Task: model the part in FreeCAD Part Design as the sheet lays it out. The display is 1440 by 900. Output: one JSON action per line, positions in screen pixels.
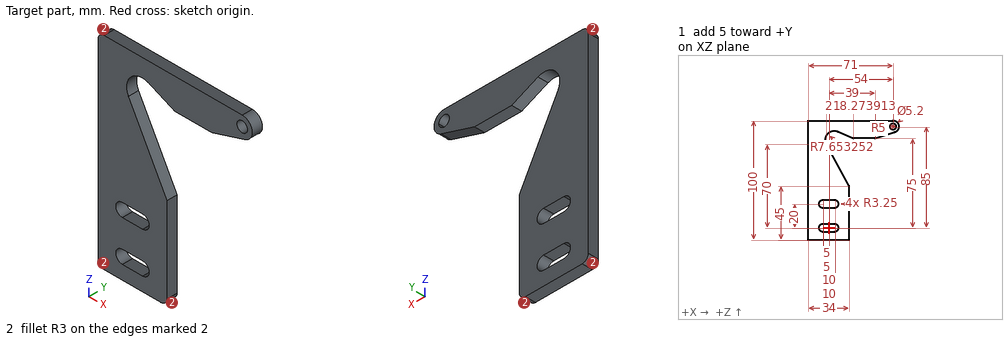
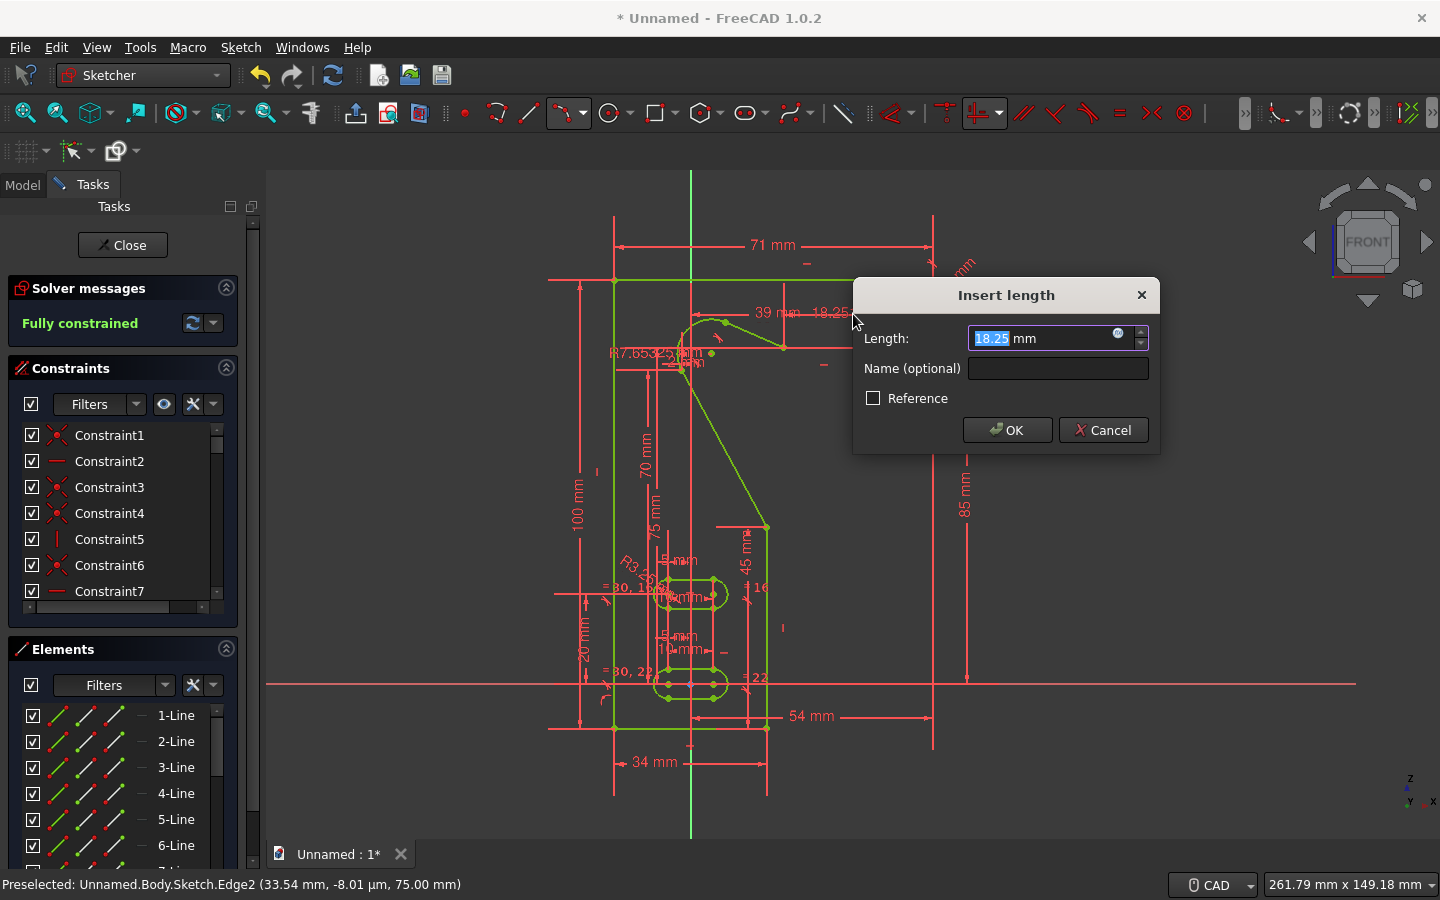
{"action": "type", "text": "18.273913"}
{"action": "key", "text": "Return"}
{"action": "key", "text": "Escape"}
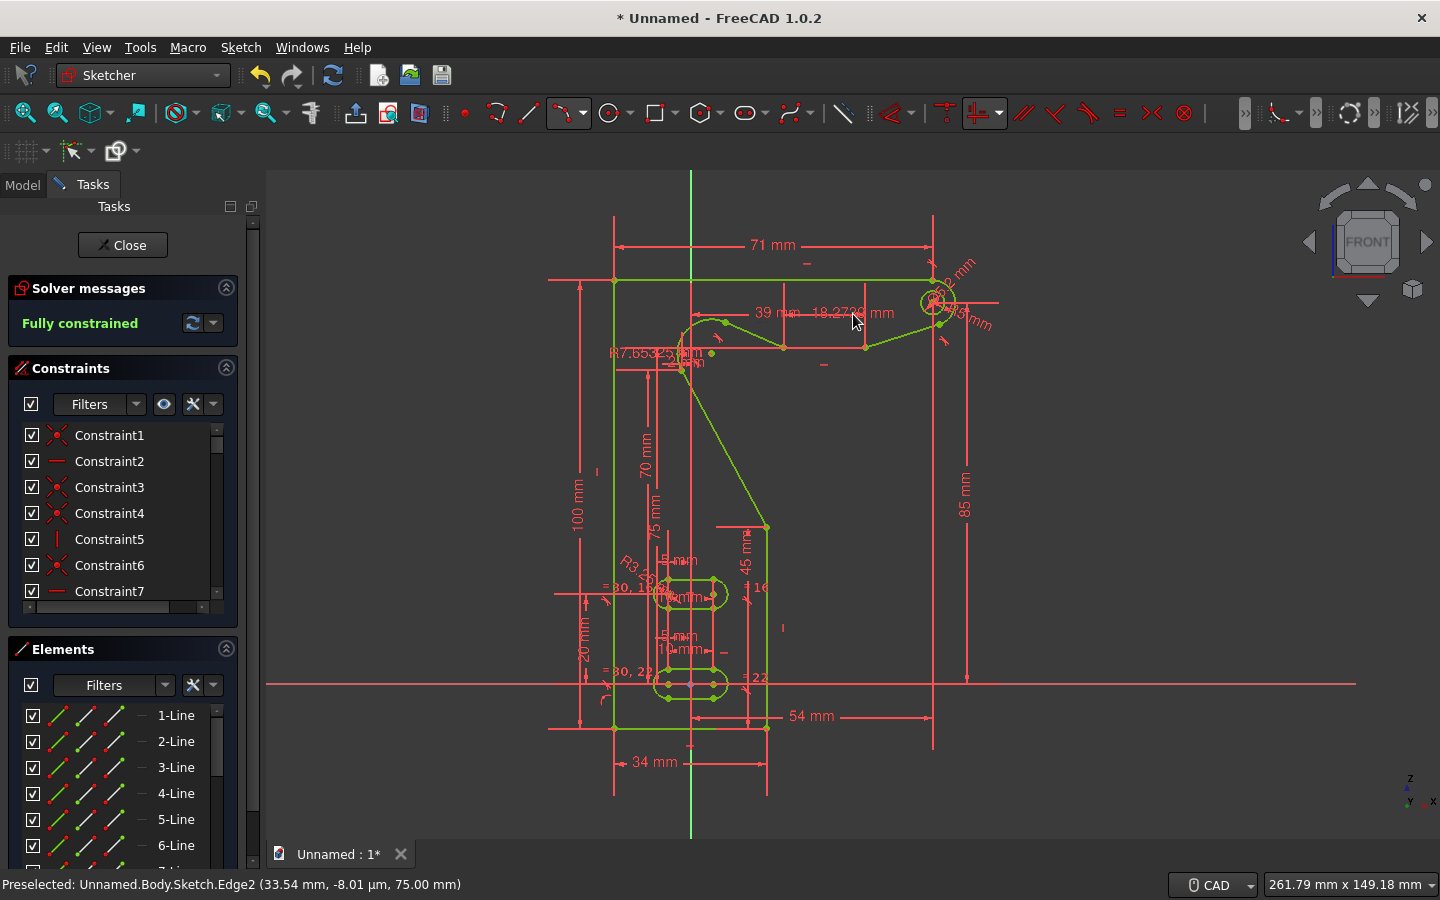
{"action": "left_click", "coordinate": [123, 245]}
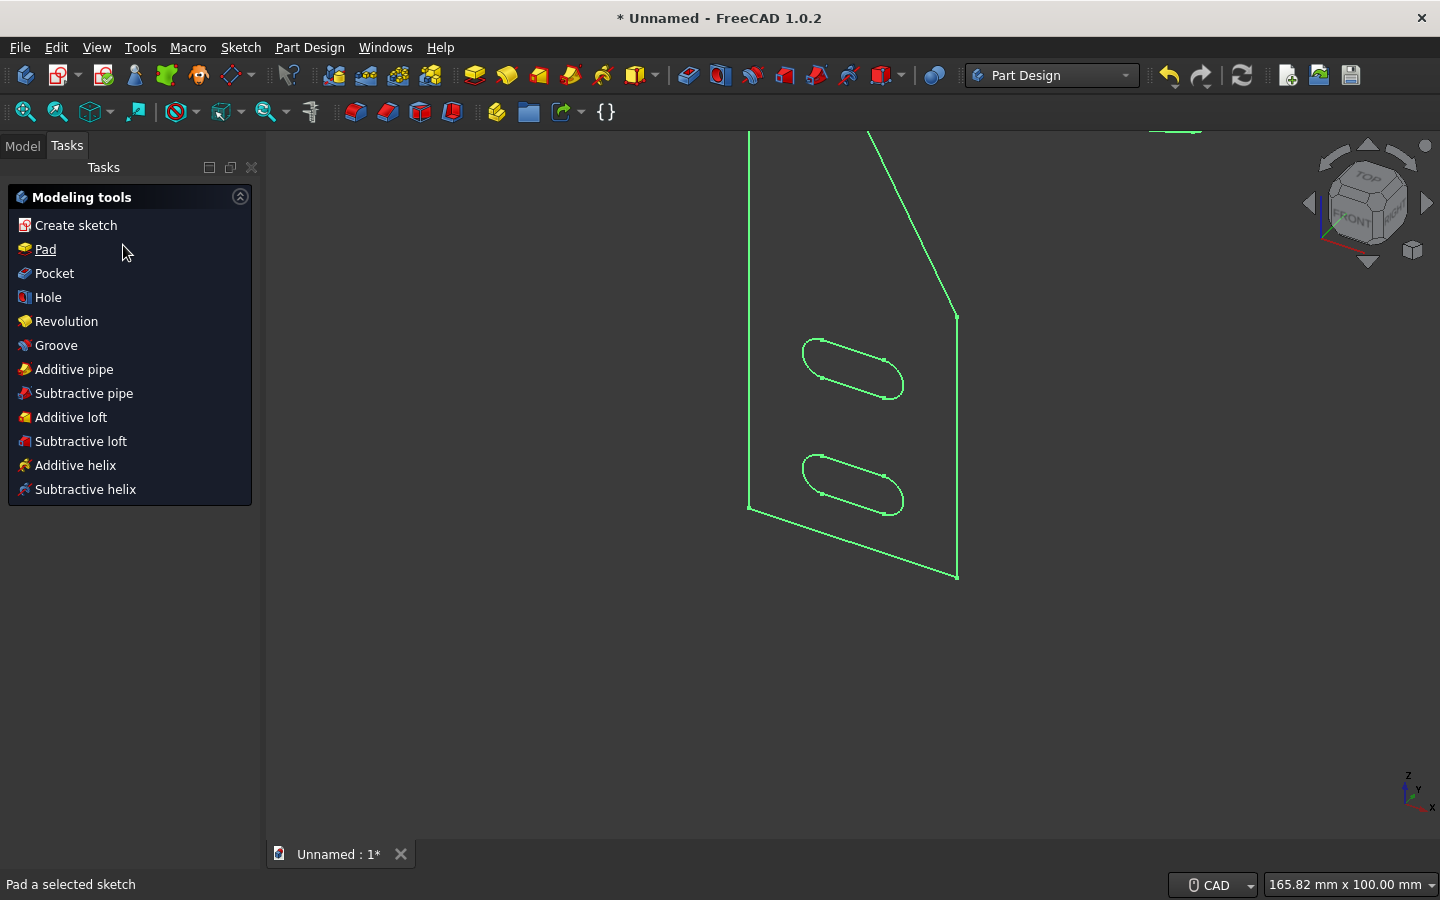
{"action": "left_click", "coordinate": [476, 76]}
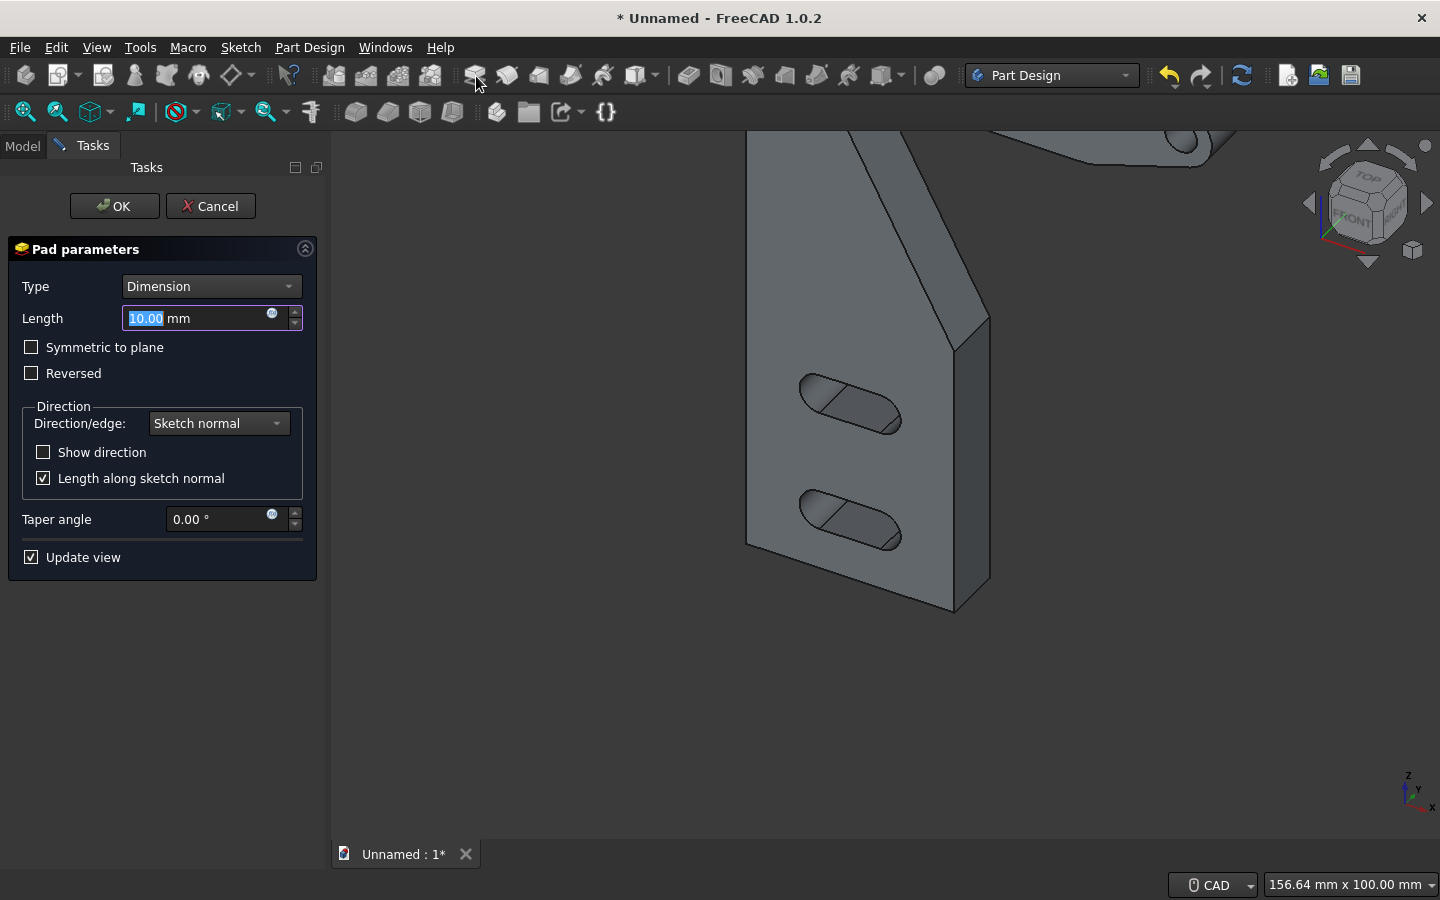
{"action": "type", "text": "5"}
{"action": "key", "text": "Tab"}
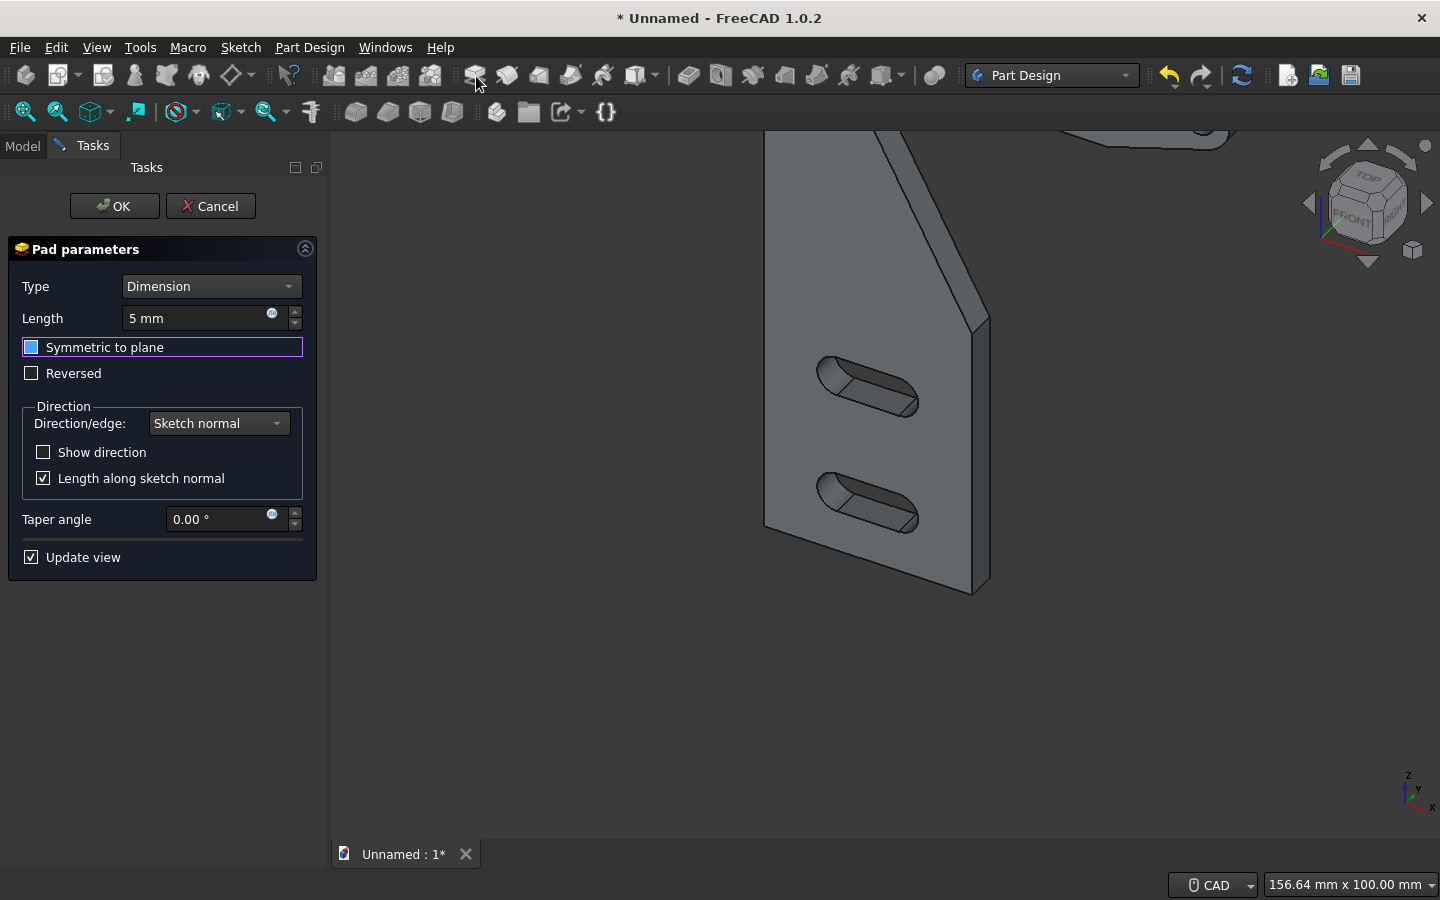
{"action": "left_click", "coordinate": [30, 373]}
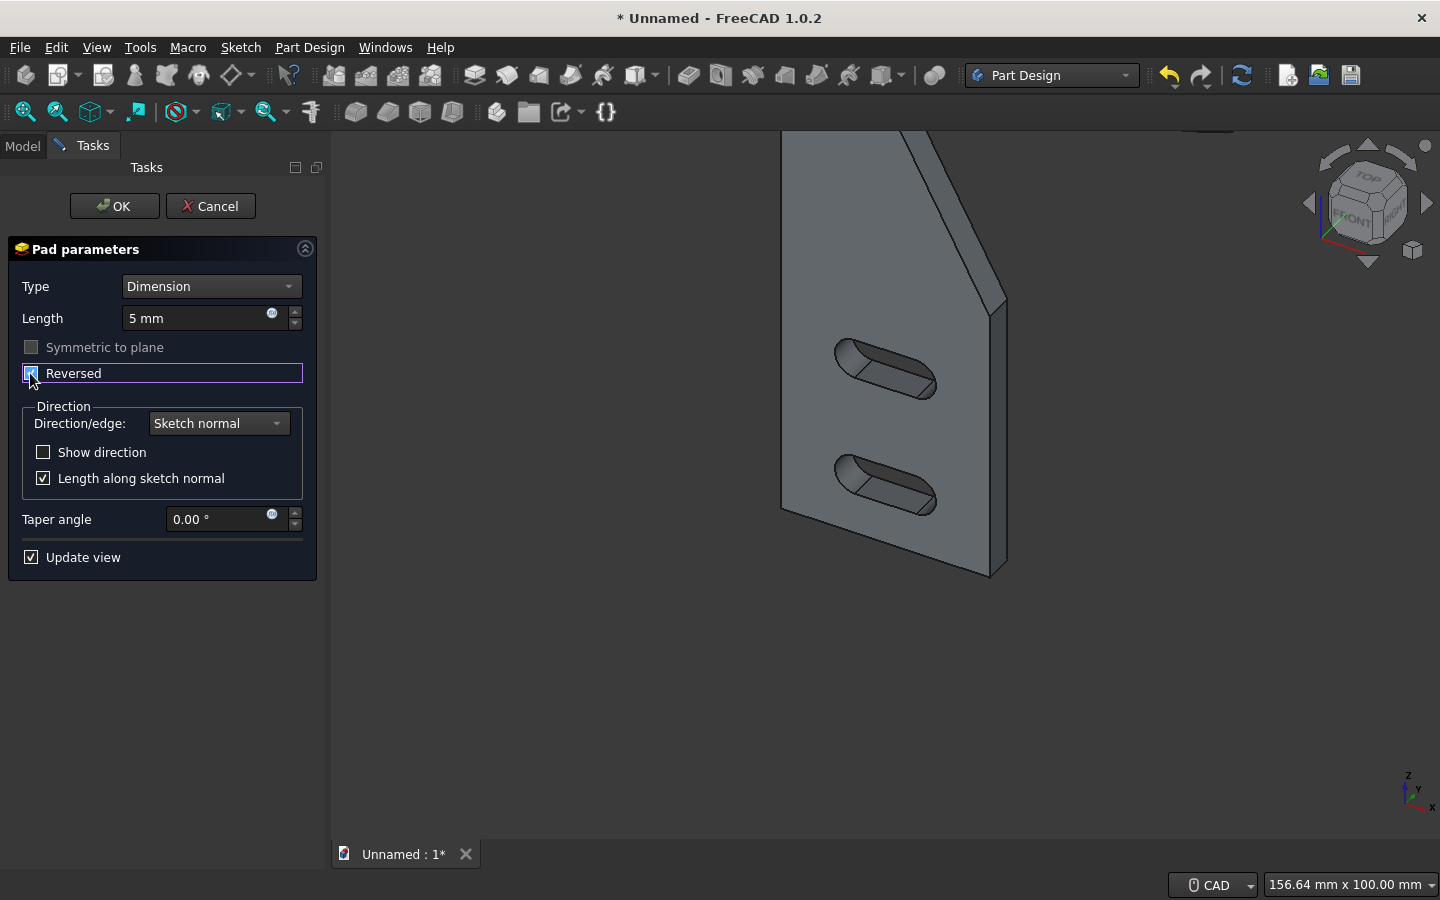
{"action": "left_click", "coordinate": [115, 206]}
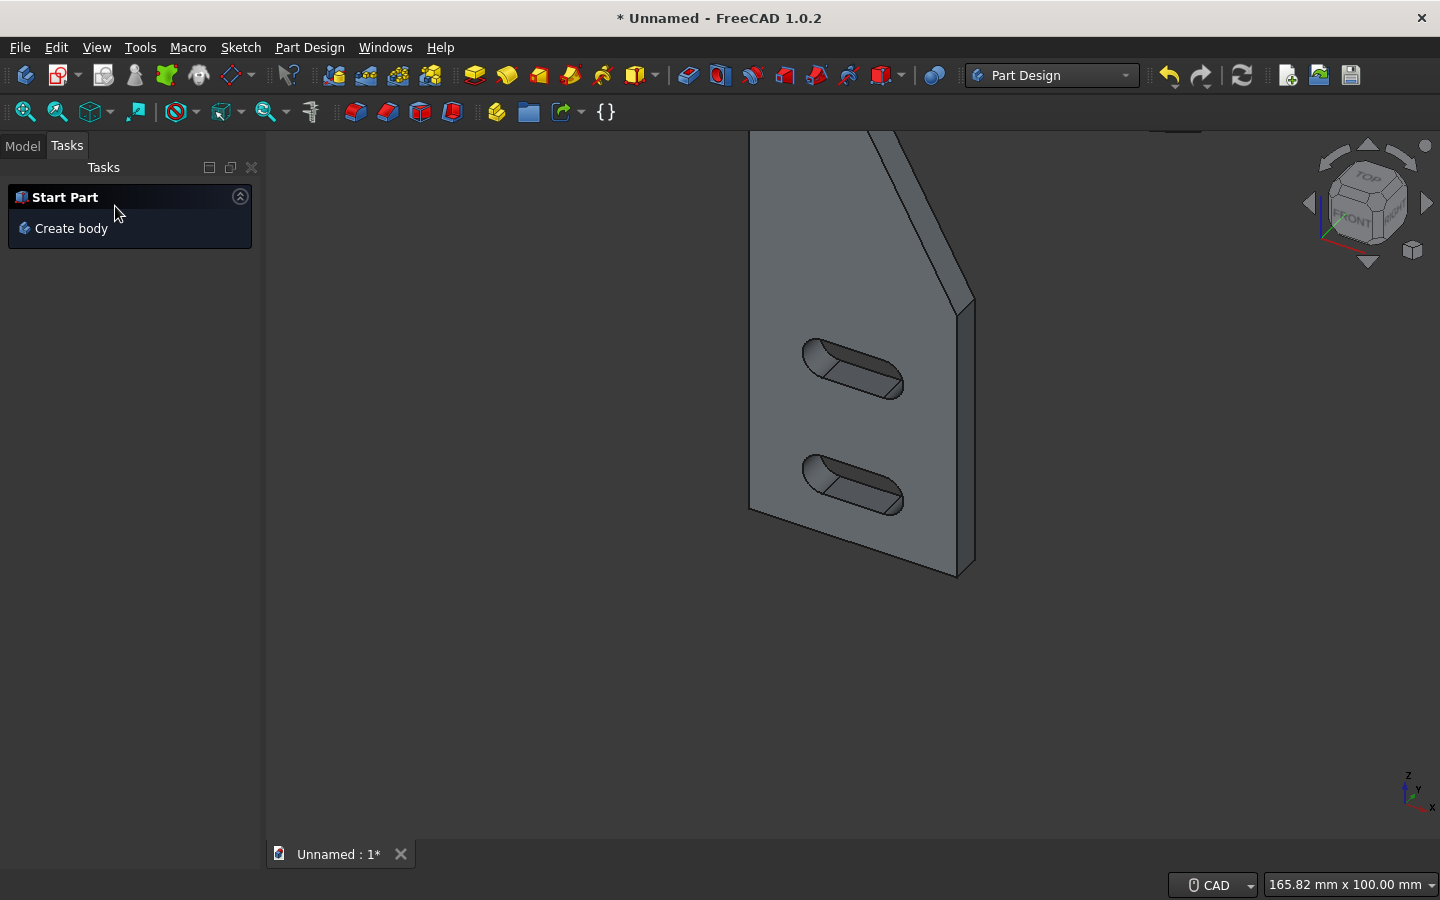
{"action": "left_click", "coordinate": [26, 112]}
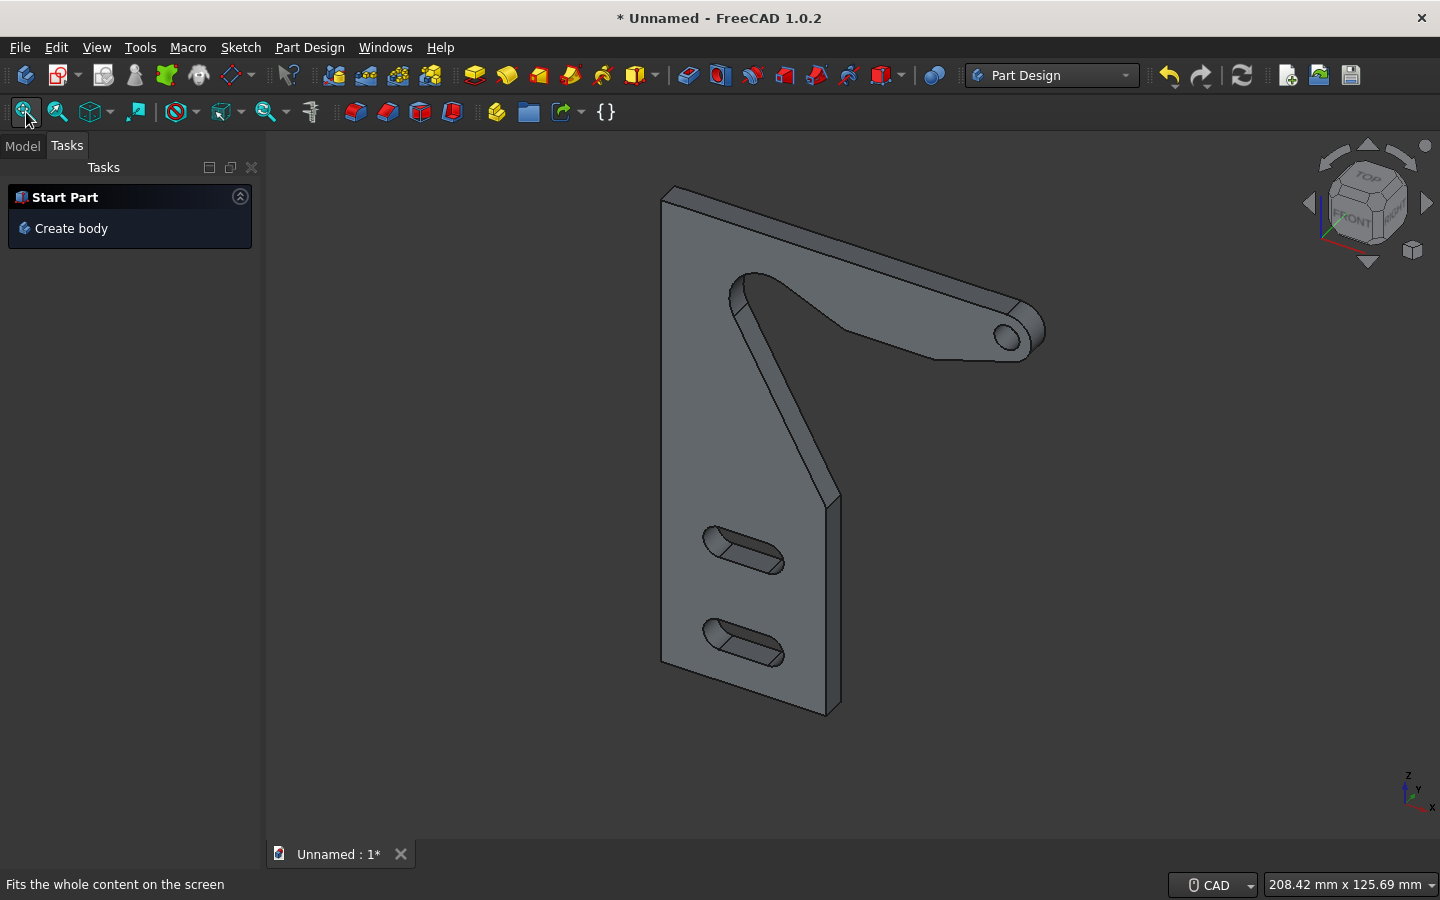
{"action": "key", "text": "0"}